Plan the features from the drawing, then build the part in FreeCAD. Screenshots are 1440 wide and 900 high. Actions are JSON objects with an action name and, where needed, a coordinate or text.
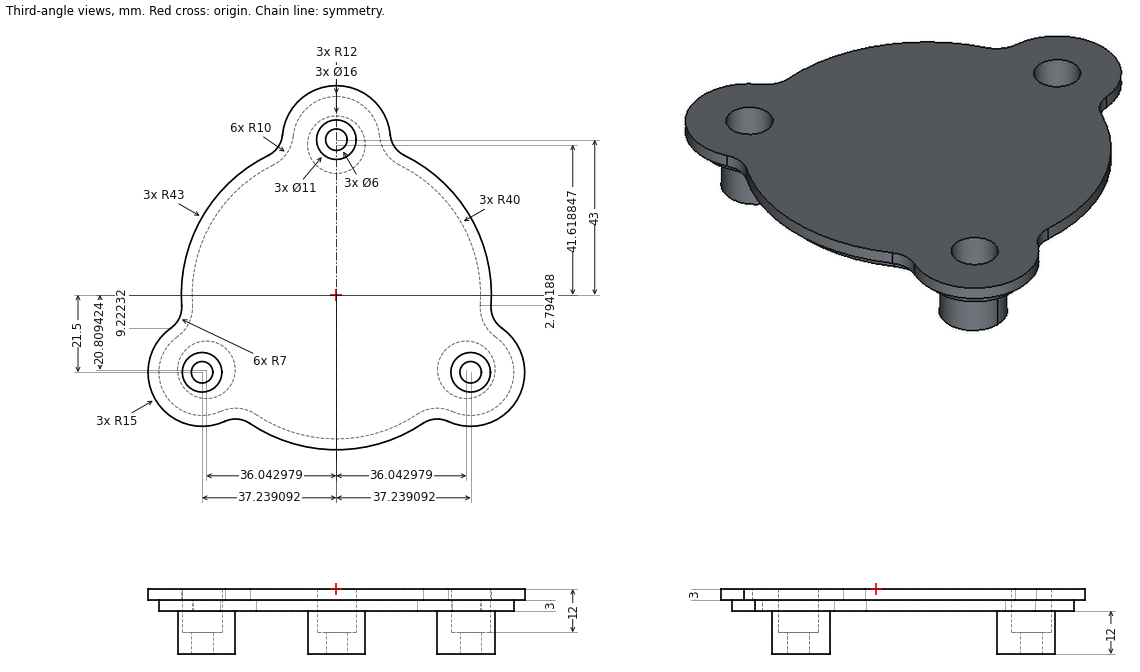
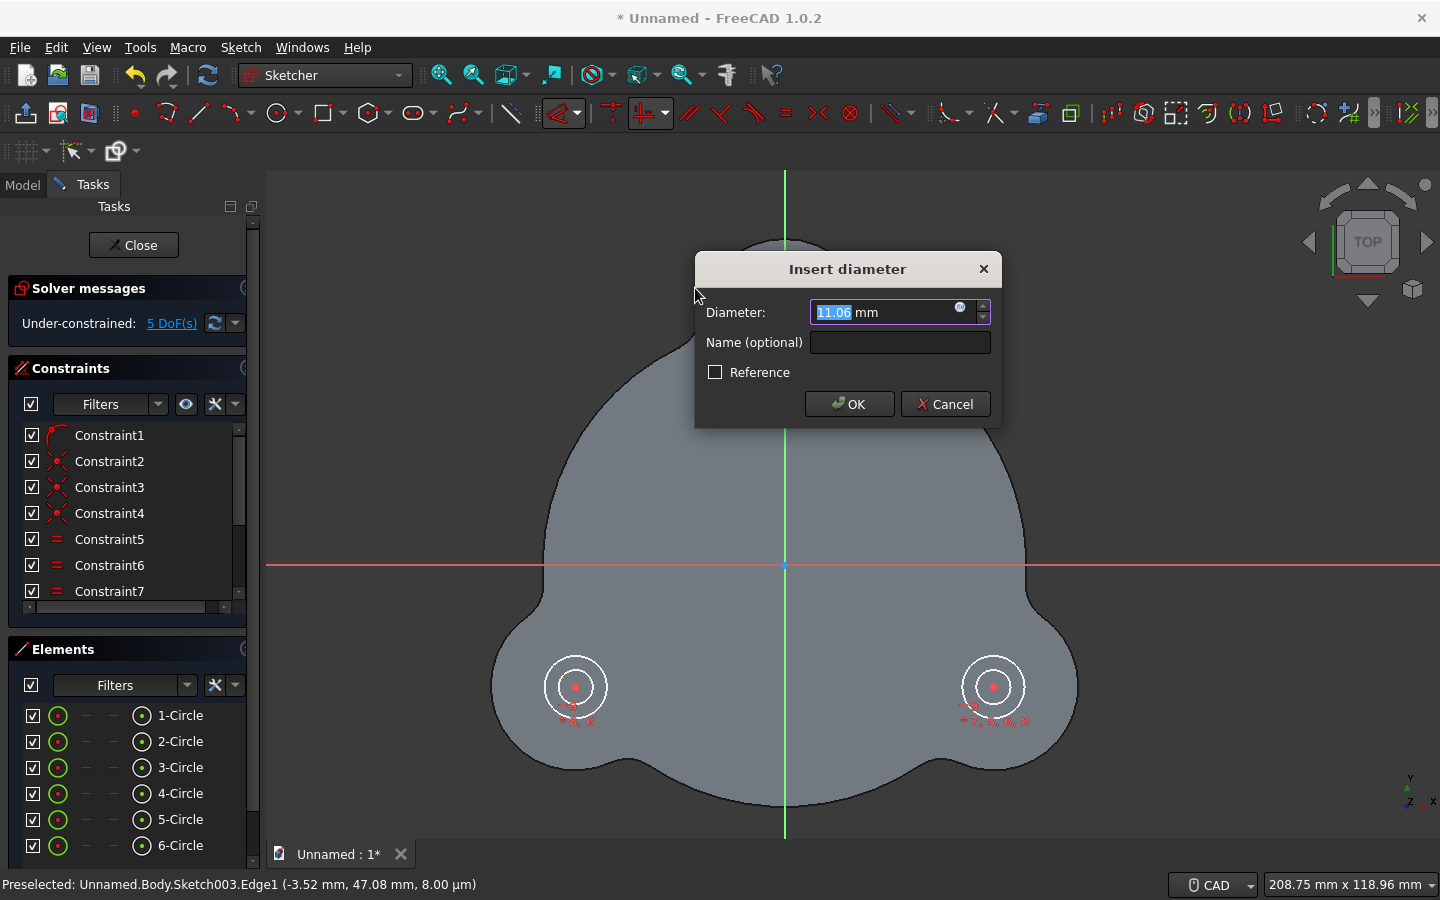
{"action": "type", "text": "11"}
{"action": "key", "text": "Return"}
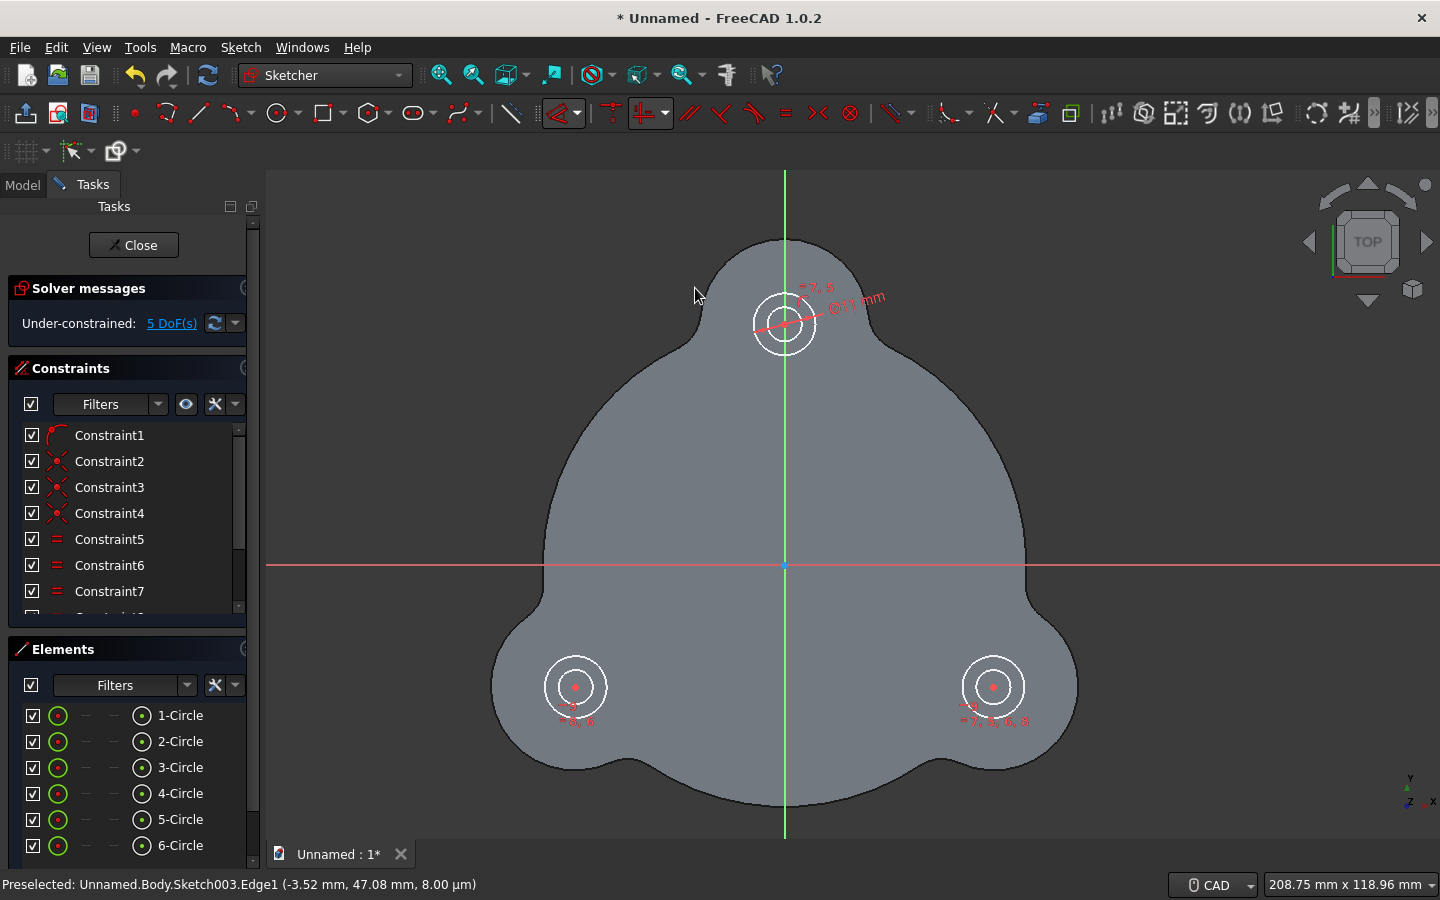
{"action": "left_click", "coordinate": [797, 312]}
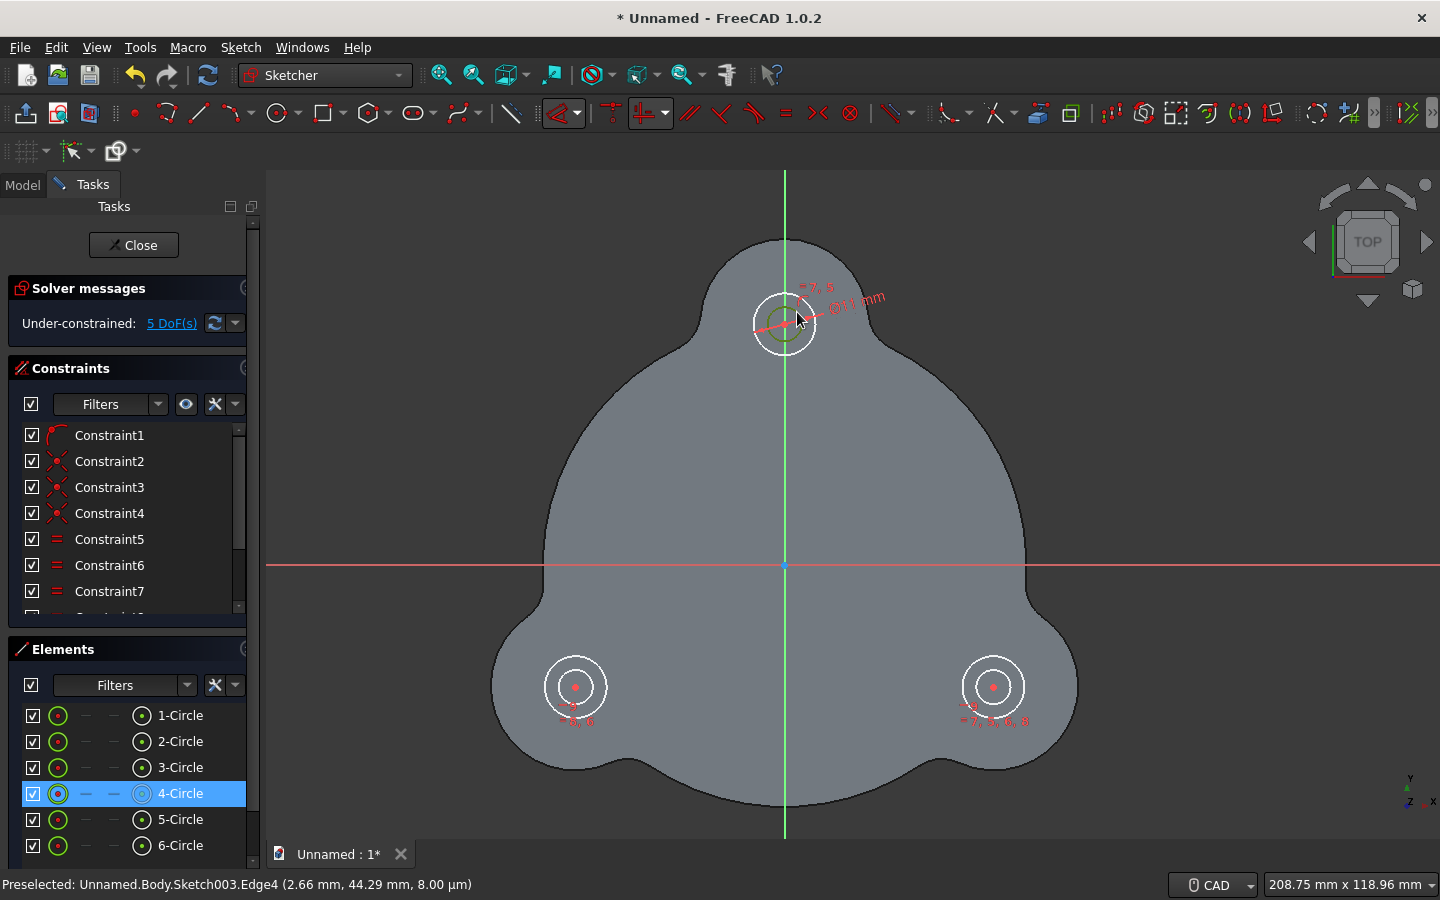
{"action": "key", "text": "k o"}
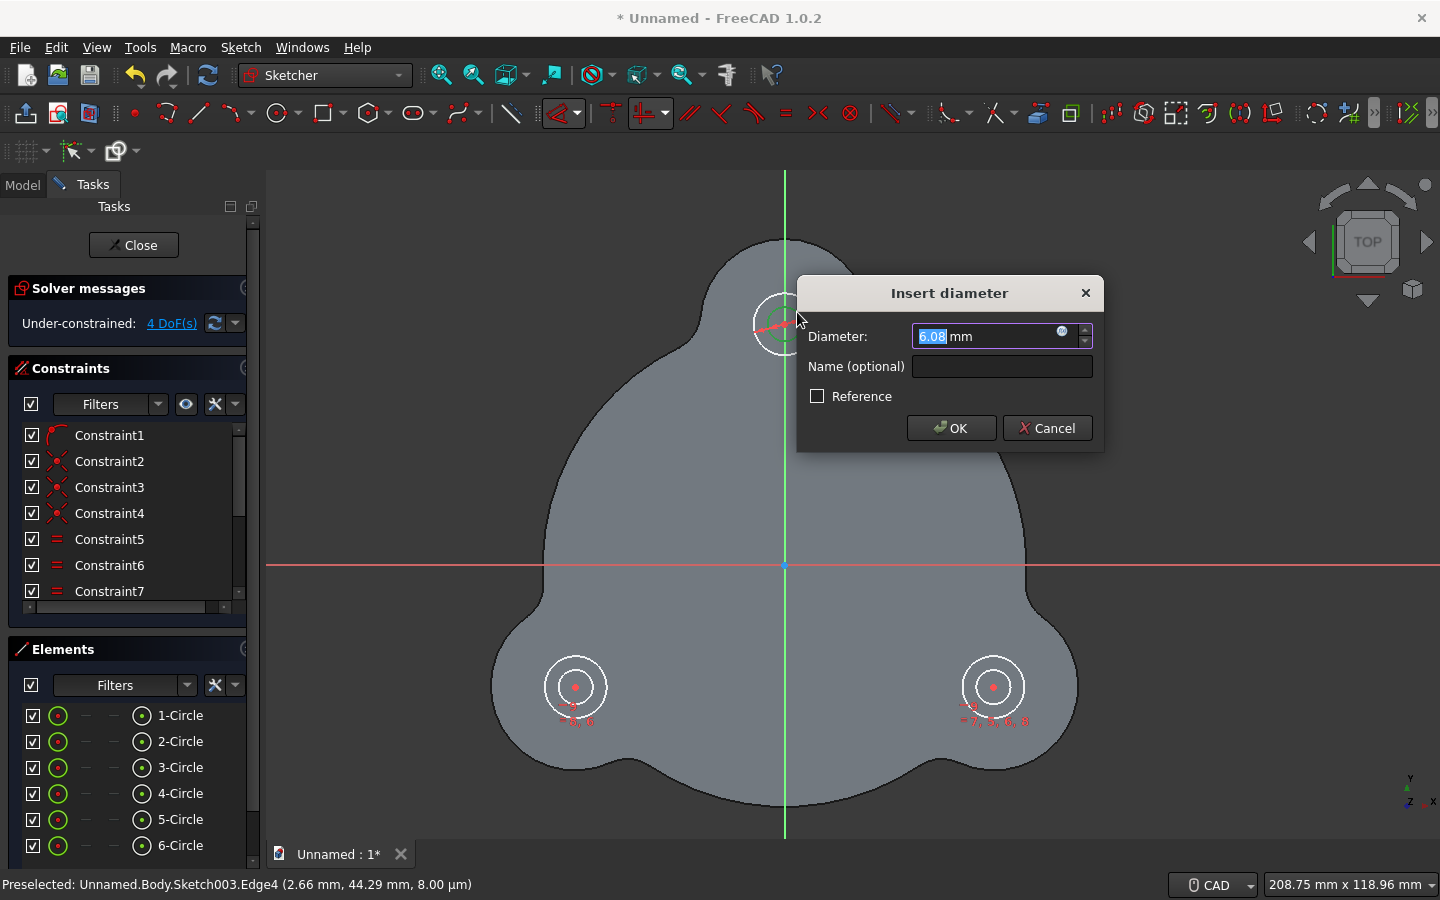
{"action": "type", "text": "6"}
{"action": "key", "text": "Return"}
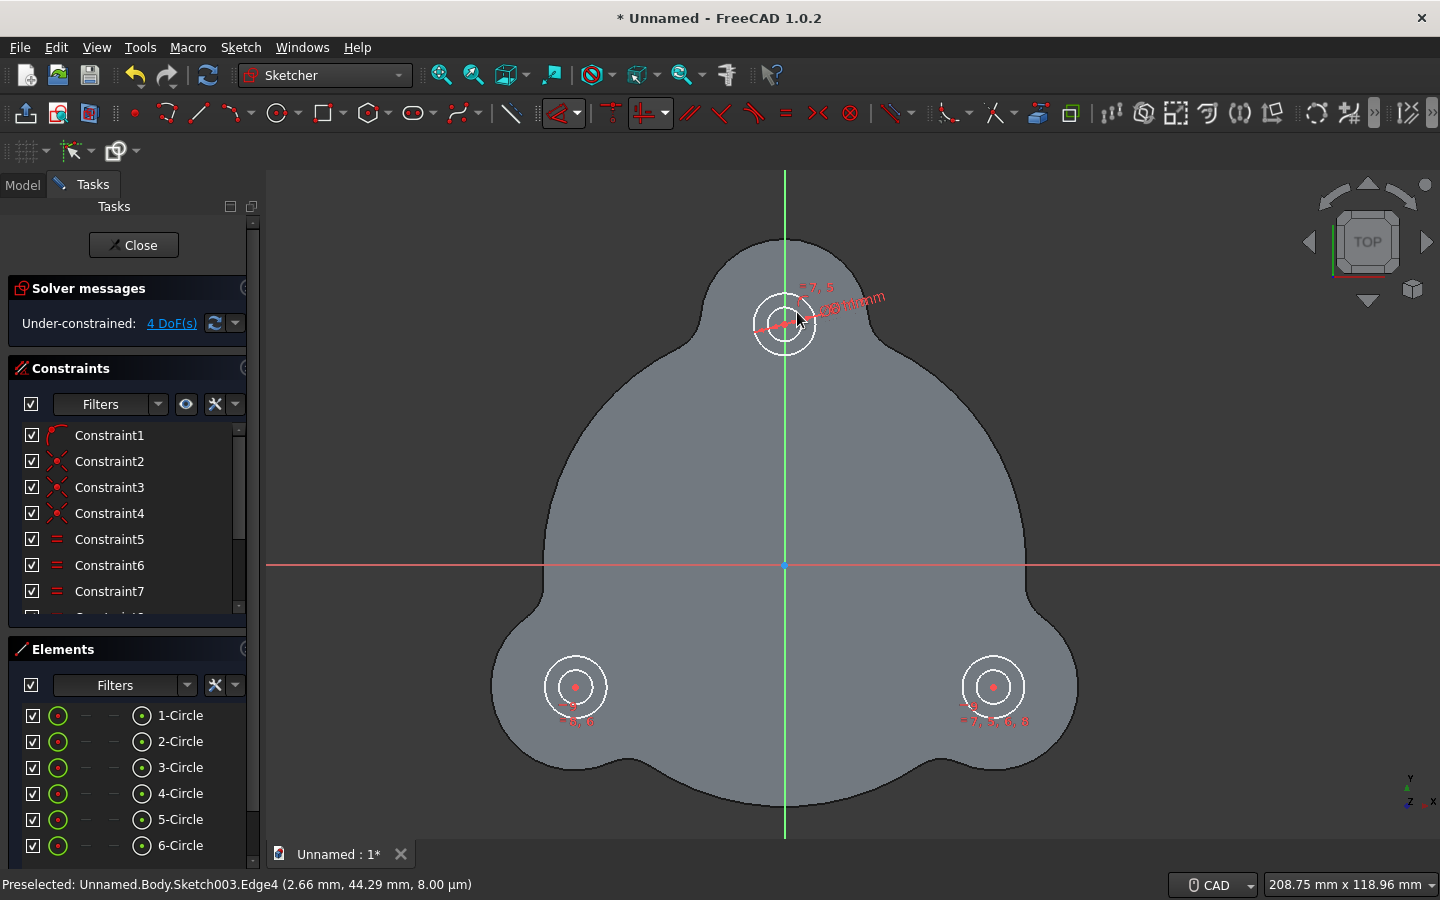
{"action": "left_click", "coordinate": [785, 324]}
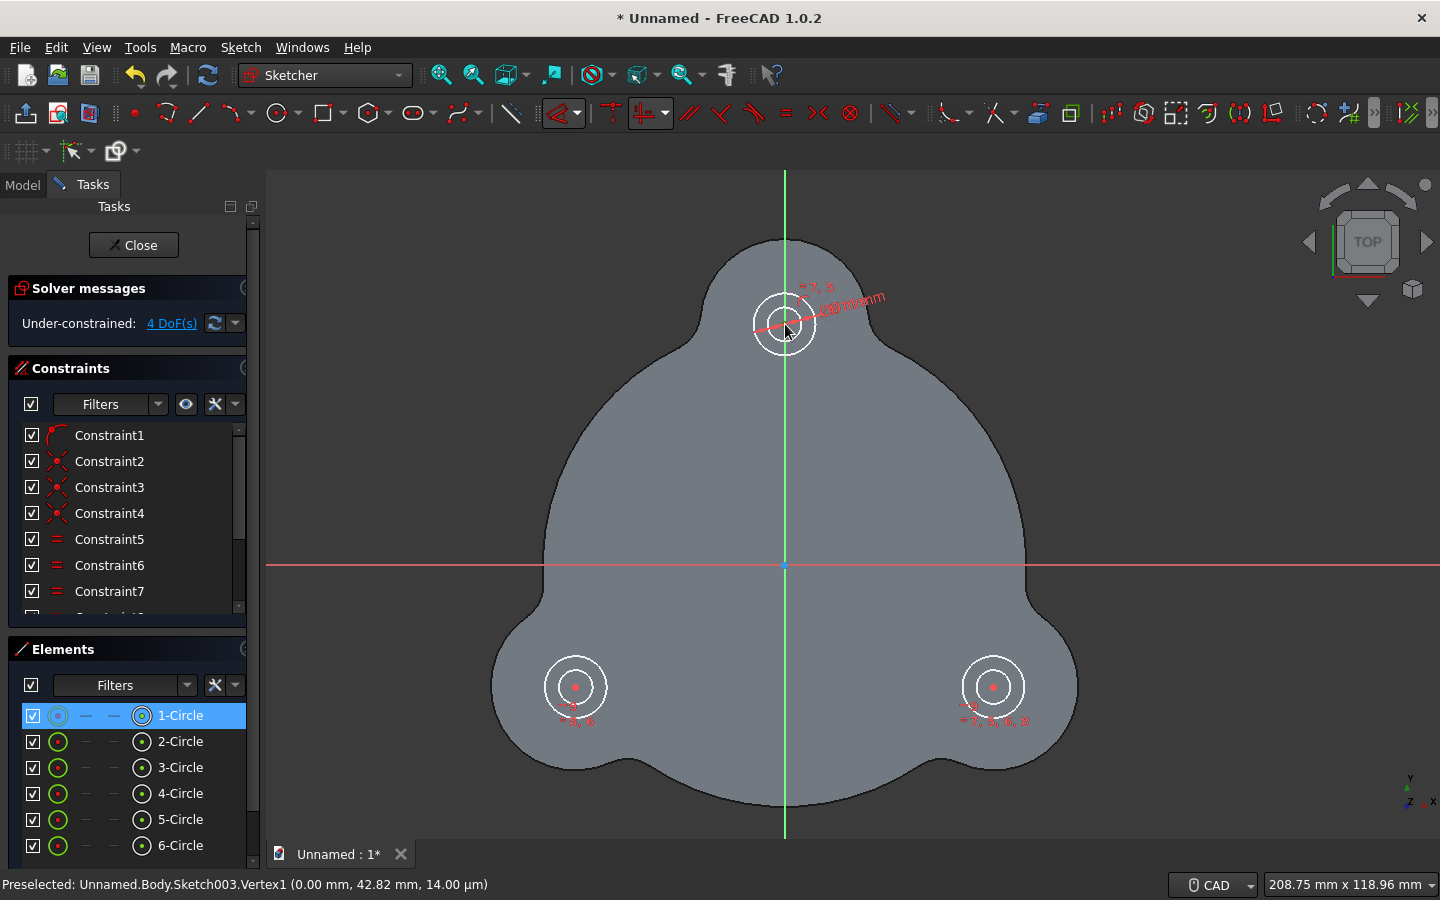
{"action": "key", "text": "i"}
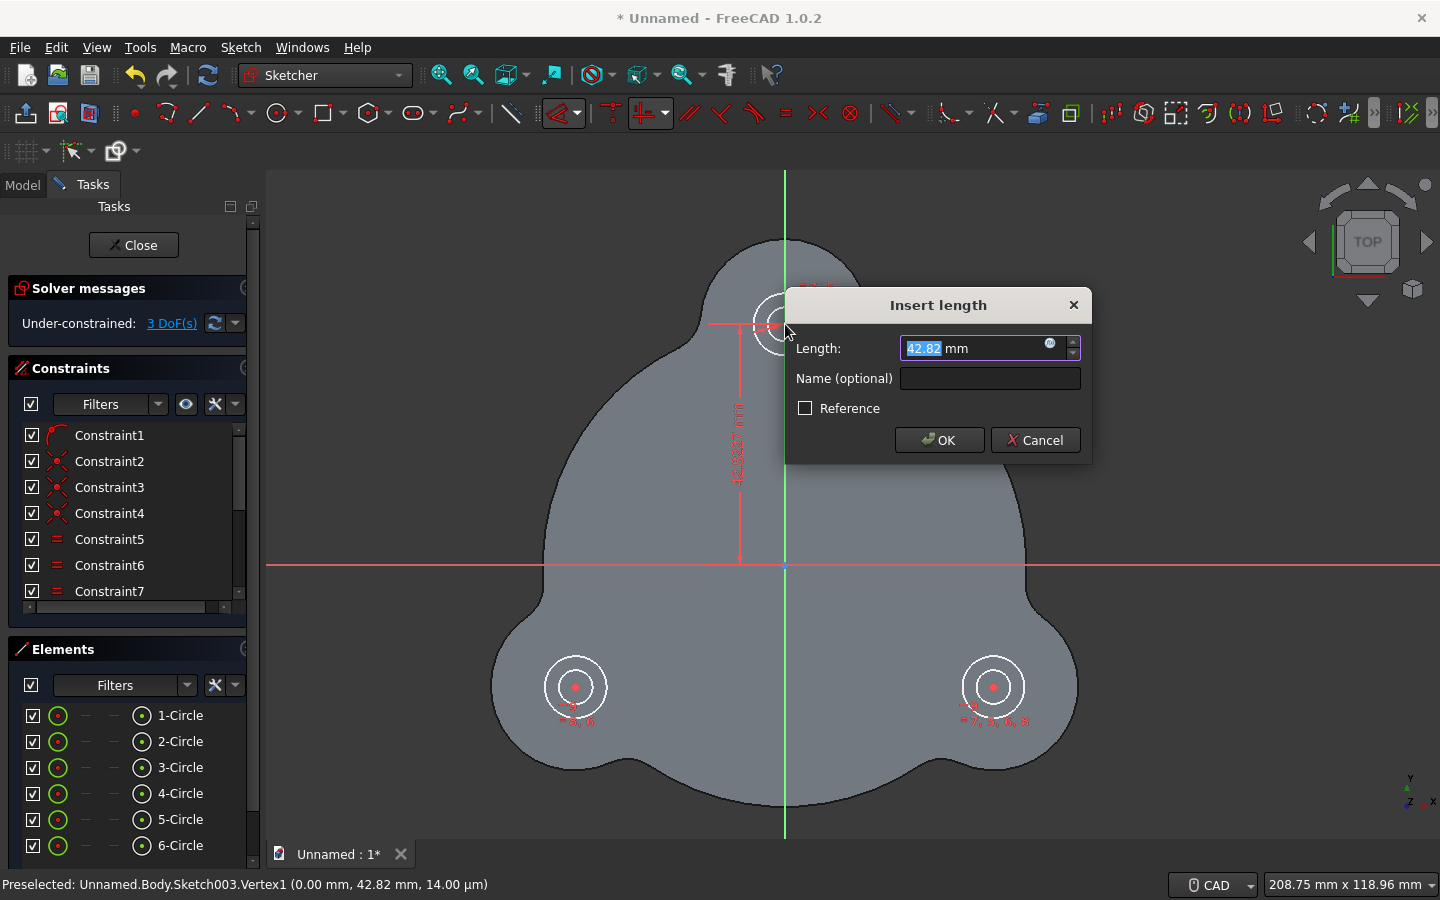
{"action": "type", "text": "43"}
{"action": "key", "text": "Return"}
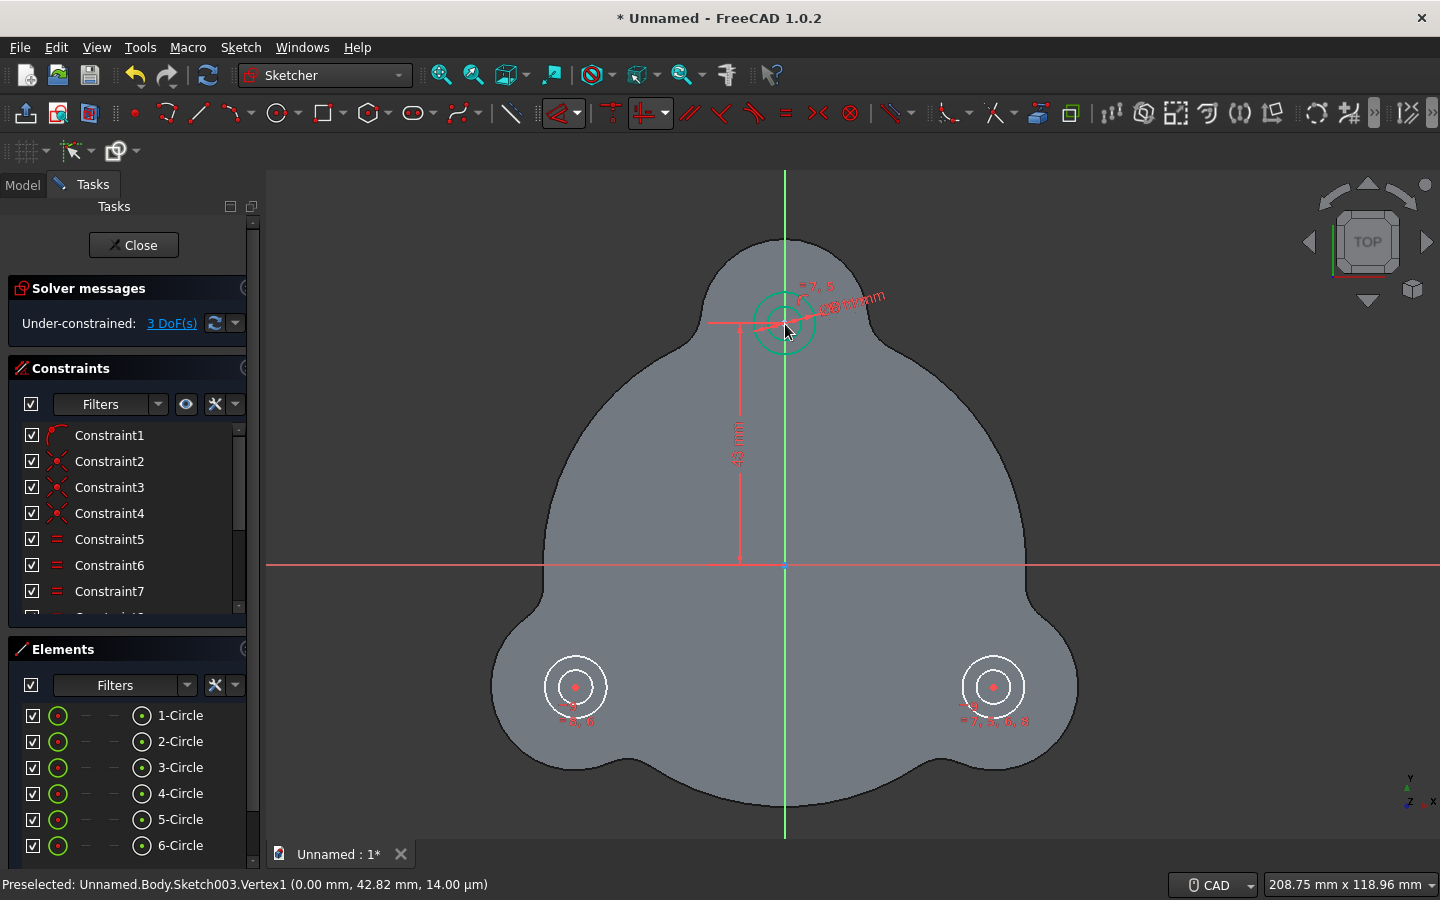
{"action": "left_click", "coordinate": [993, 687]}